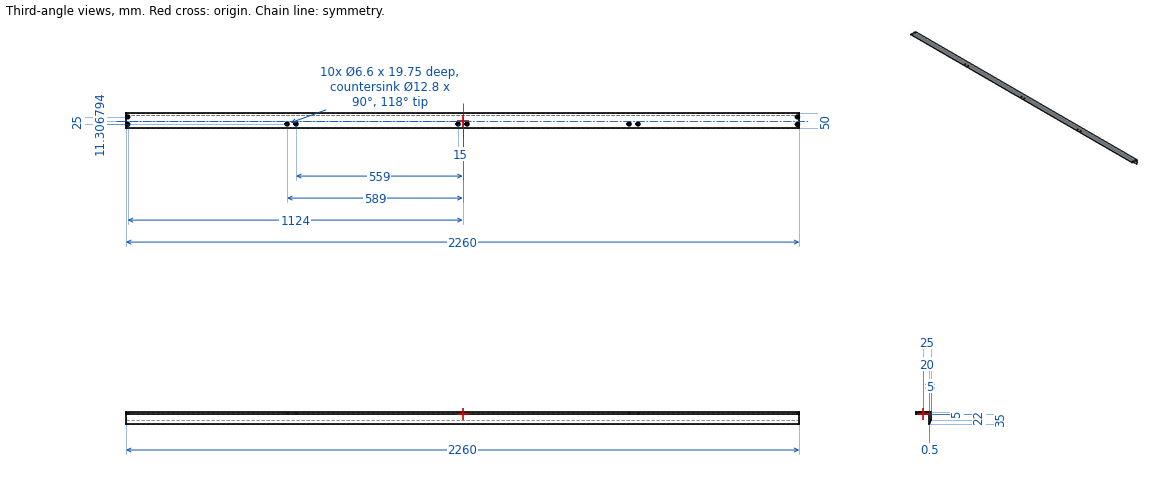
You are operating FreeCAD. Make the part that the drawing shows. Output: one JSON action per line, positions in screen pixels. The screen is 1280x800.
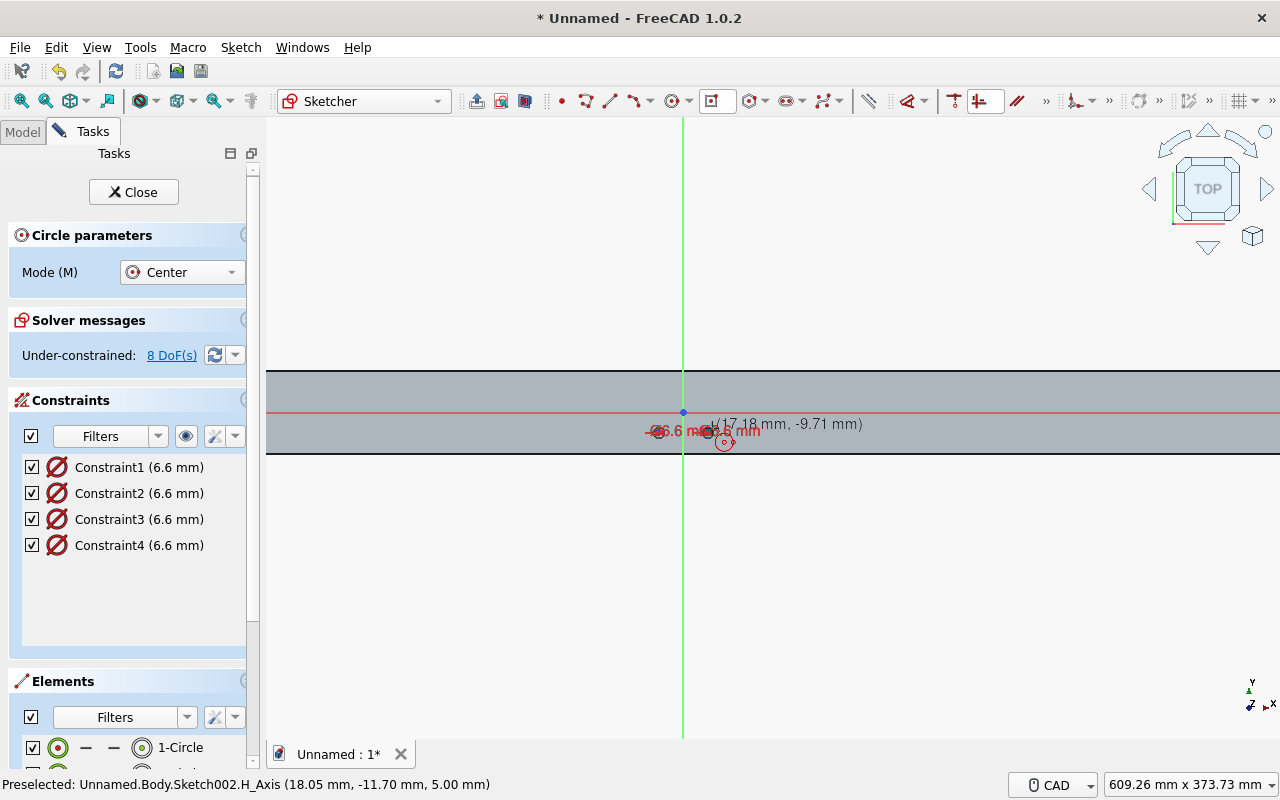
{"action": "scroll", "coordinate": [709, 431], "scroll_direction": "down", "scroll_amount": 9}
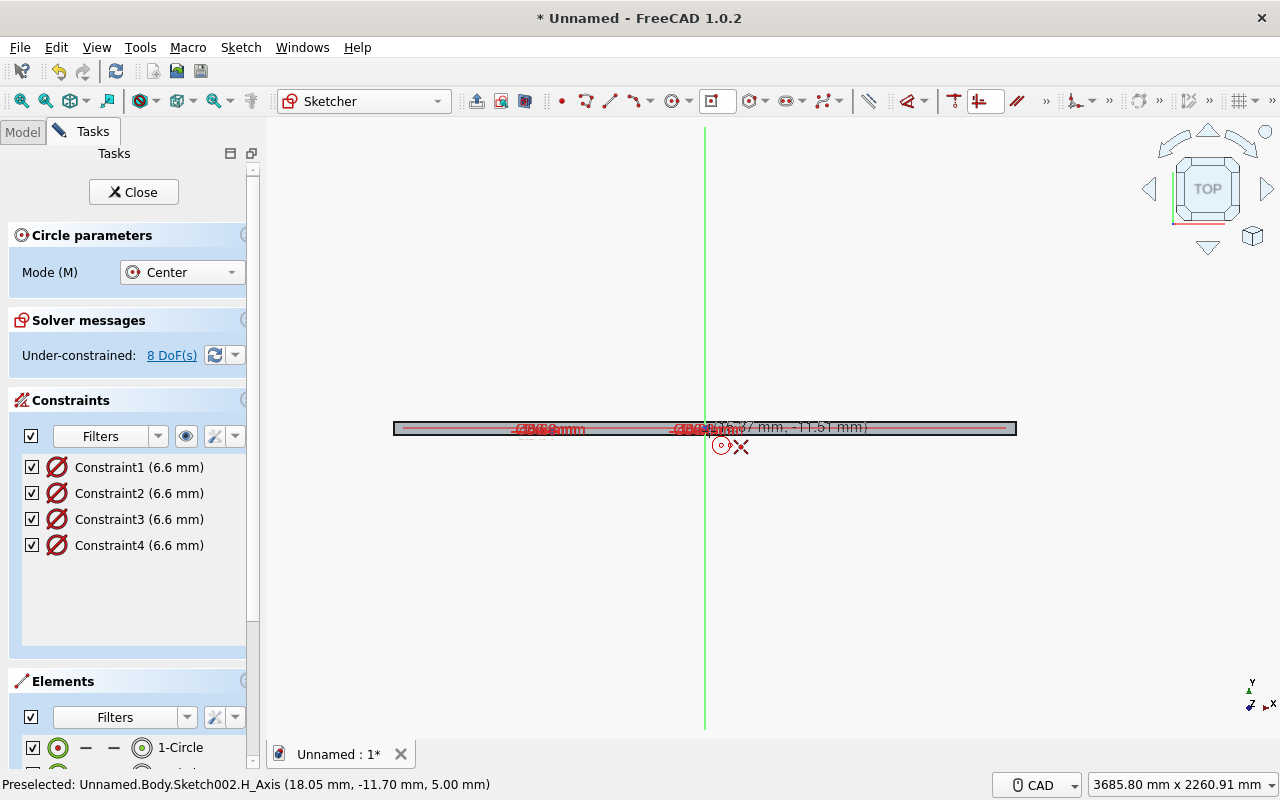
{"action": "scroll", "coordinate": [859, 432], "scroll_direction": "up", "scroll_amount": 17}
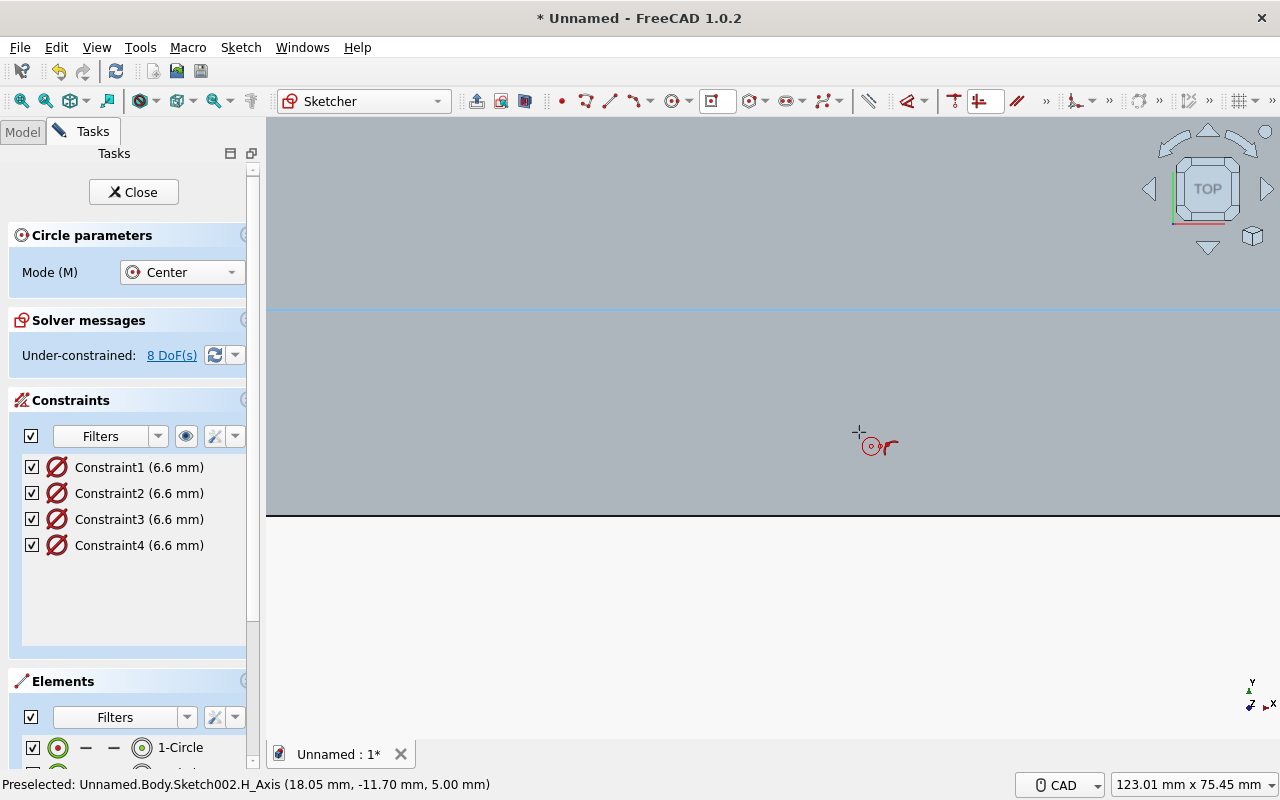
{"action": "scroll", "coordinate": [895, 433], "scroll_direction": "down", "scroll_amount": 16}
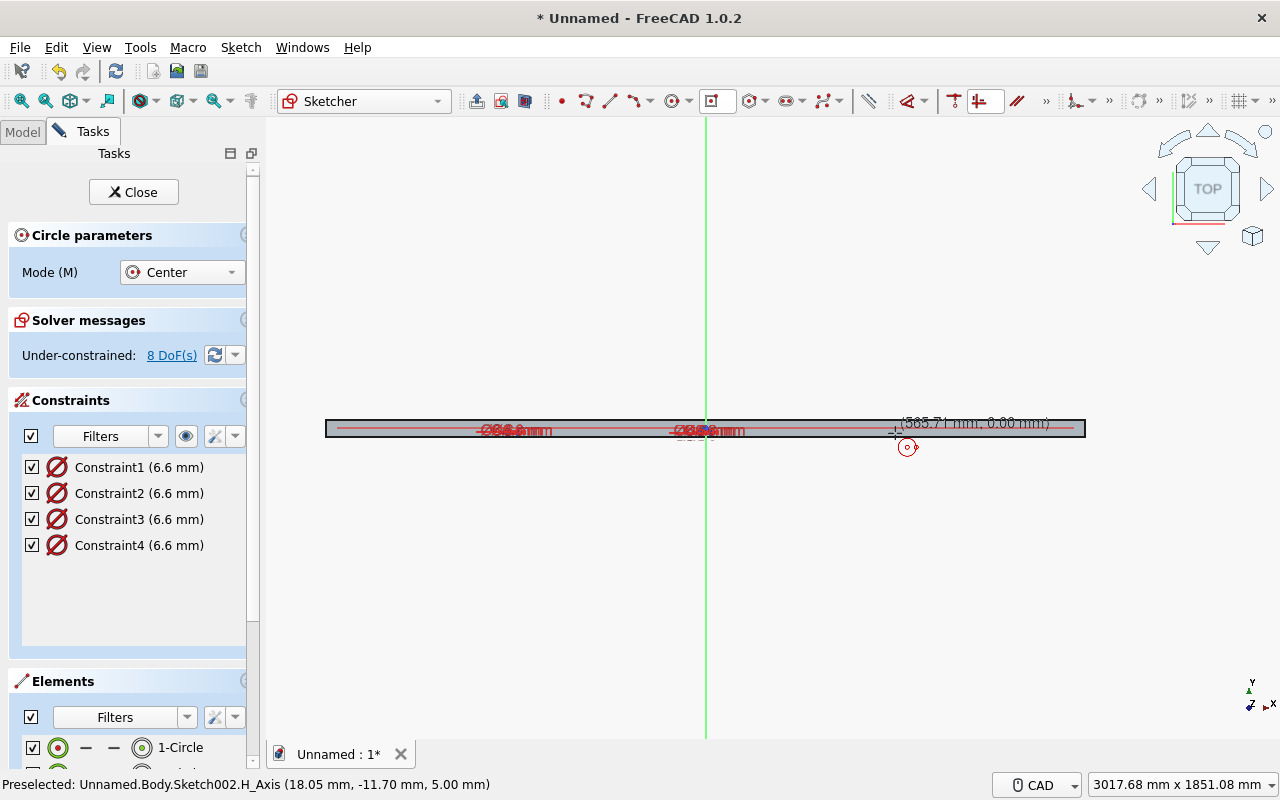
{"action": "scroll", "coordinate": [893, 432], "scroll_direction": "up", "scroll_amount": 8}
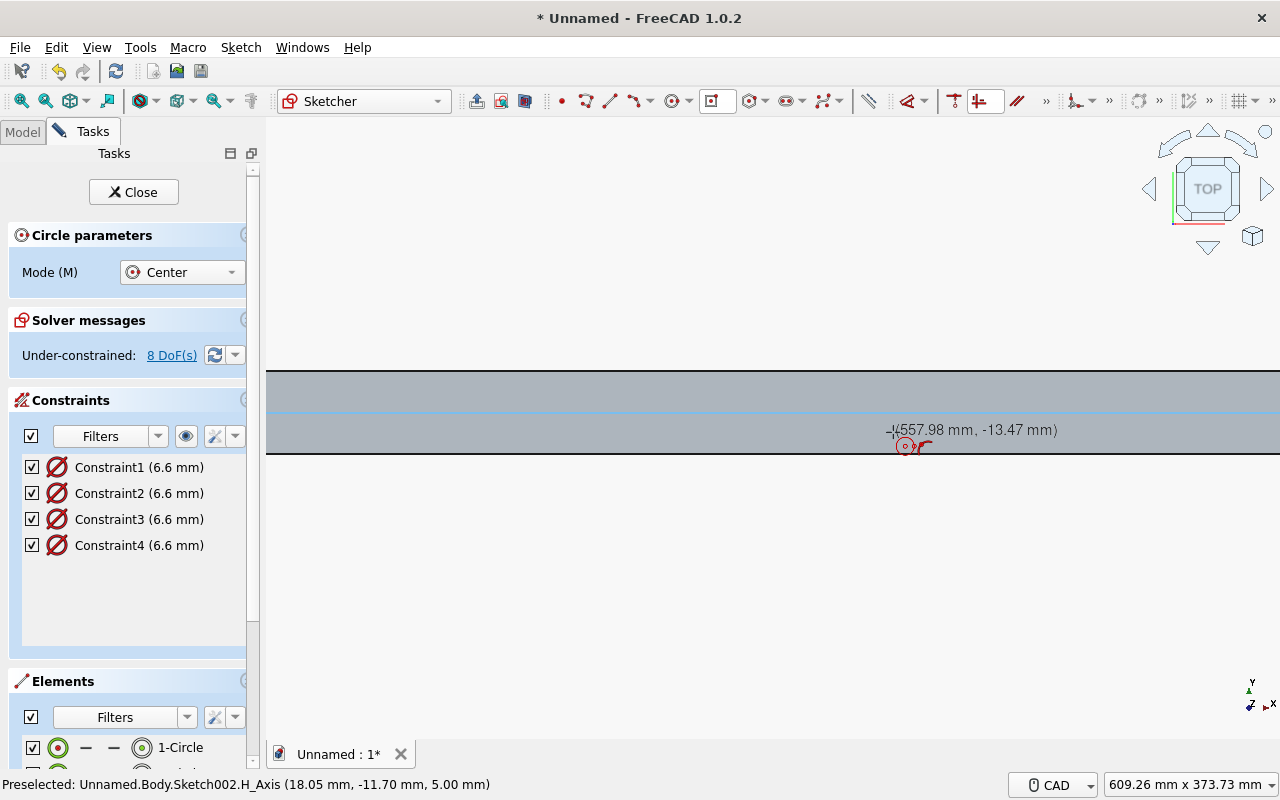
{"action": "left_click", "coordinate": [892, 431]}
{"action": "mouse_move", "coordinate": [896, 427]}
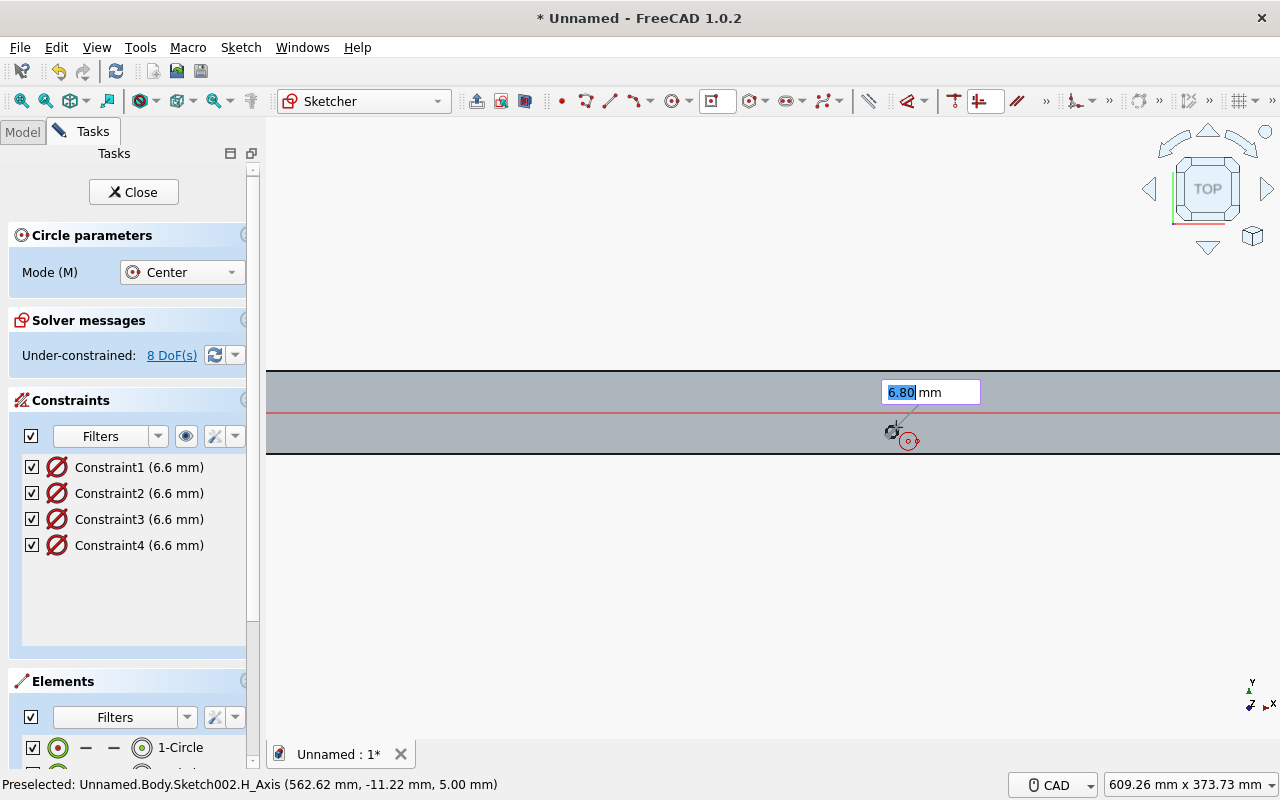
{"action": "type", "text": "6.6"}
{"action": "key", "text": "Return"}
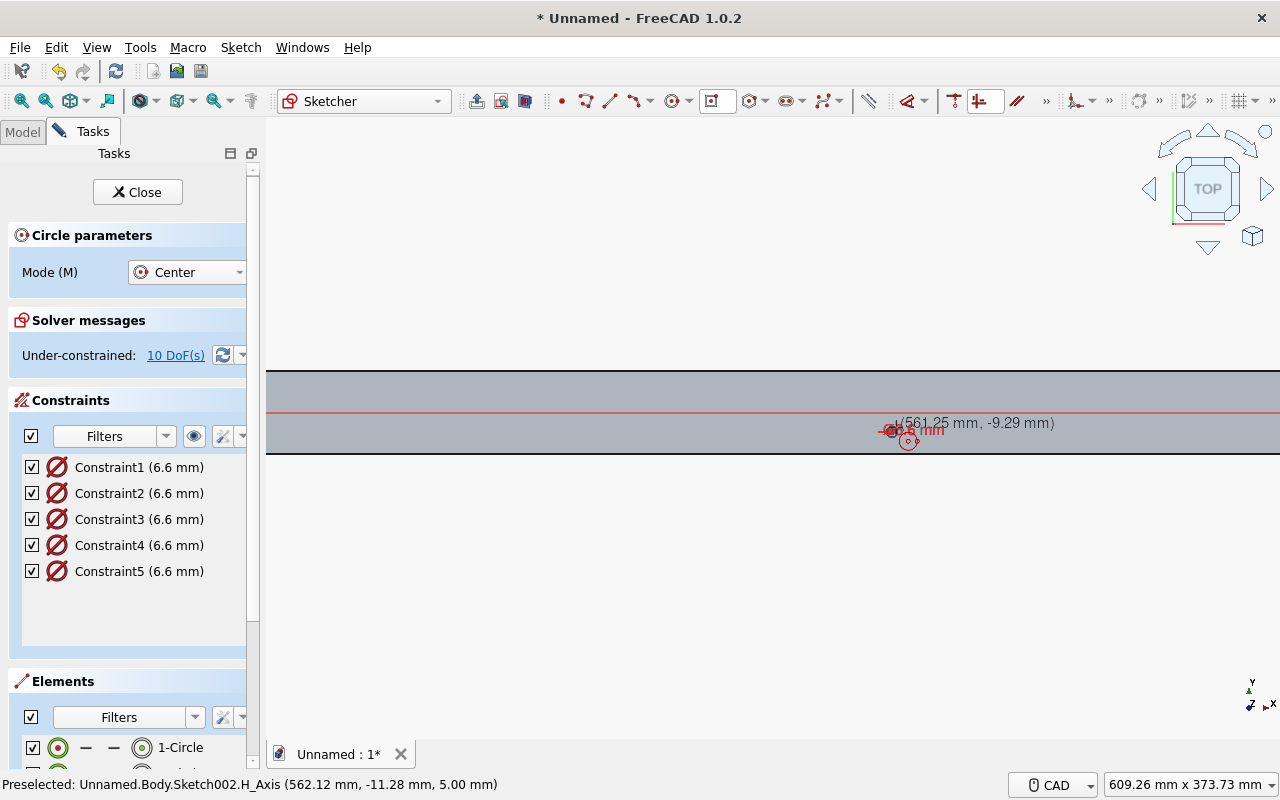
{"action": "scroll", "coordinate": [942, 431], "scroll_direction": "up", "scroll_amount": 8}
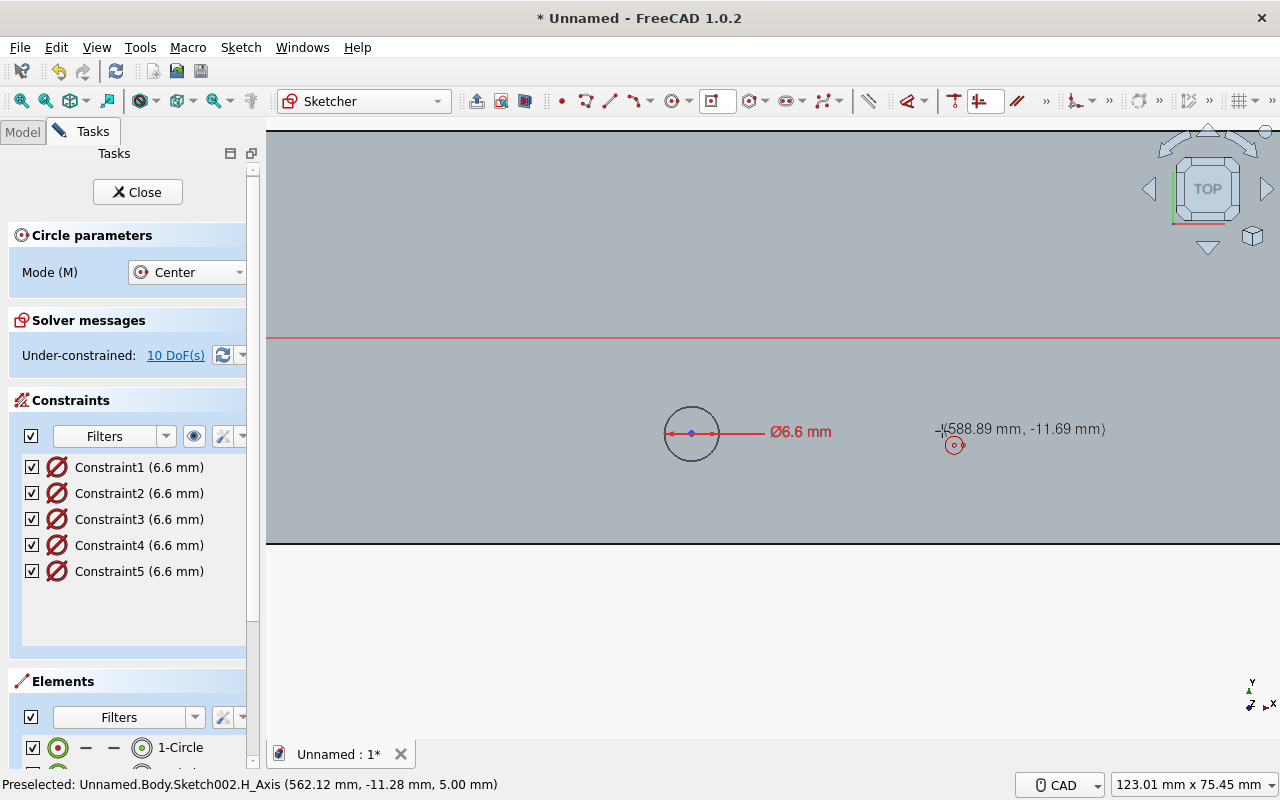
{"action": "scroll", "coordinate": [901, 432], "scroll_direction": "down", "scroll_amount": 16}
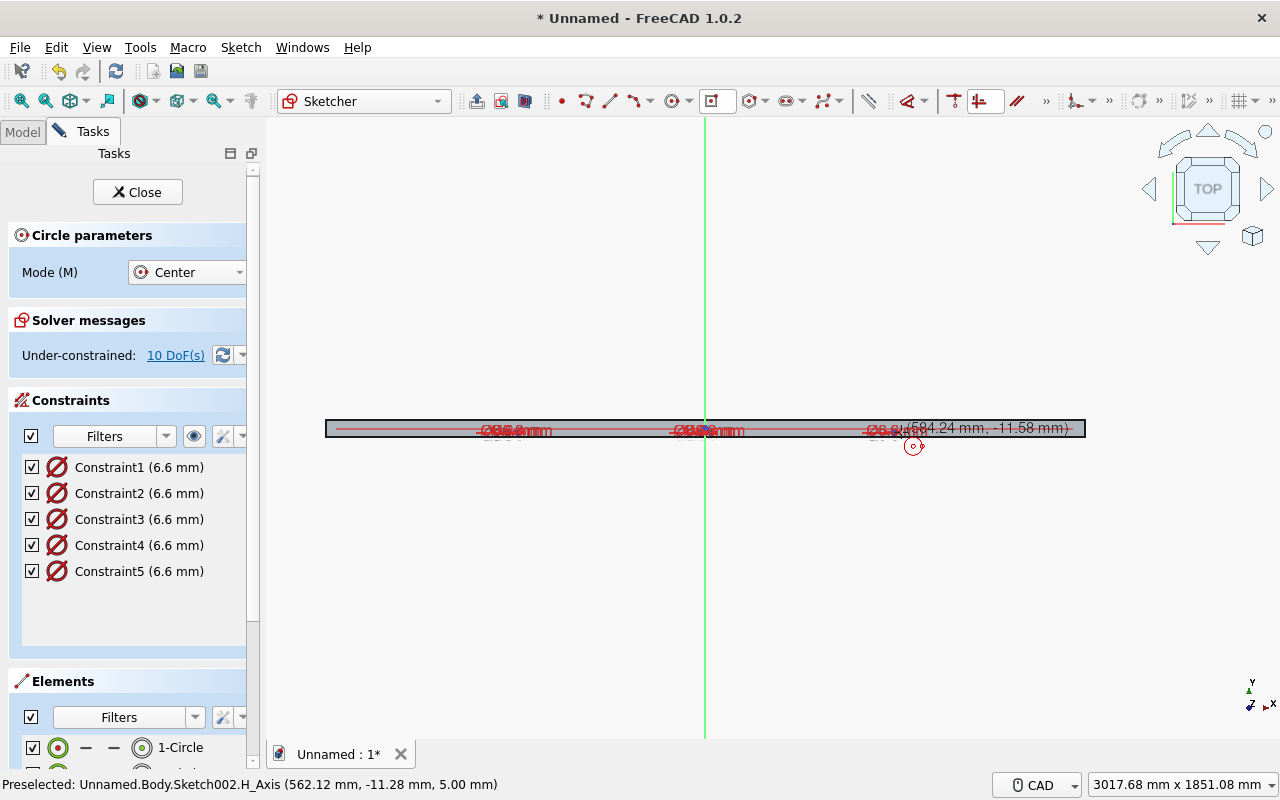
{"action": "scroll", "coordinate": [903, 432], "scroll_direction": "up", "scroll_amount": 8}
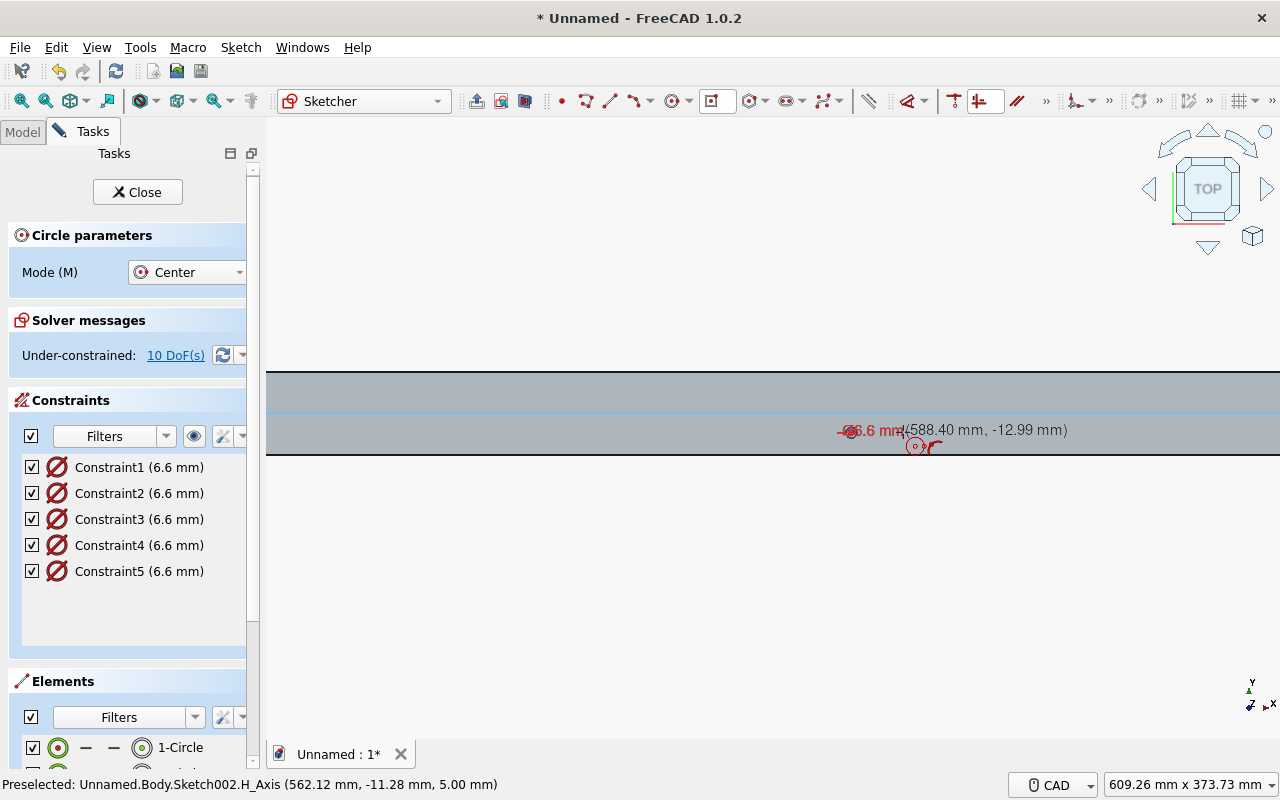
{"action": "left_click", "coordinate": [902, 432]}
{"action": "mouse_move", "coordinate": [905, 428]}